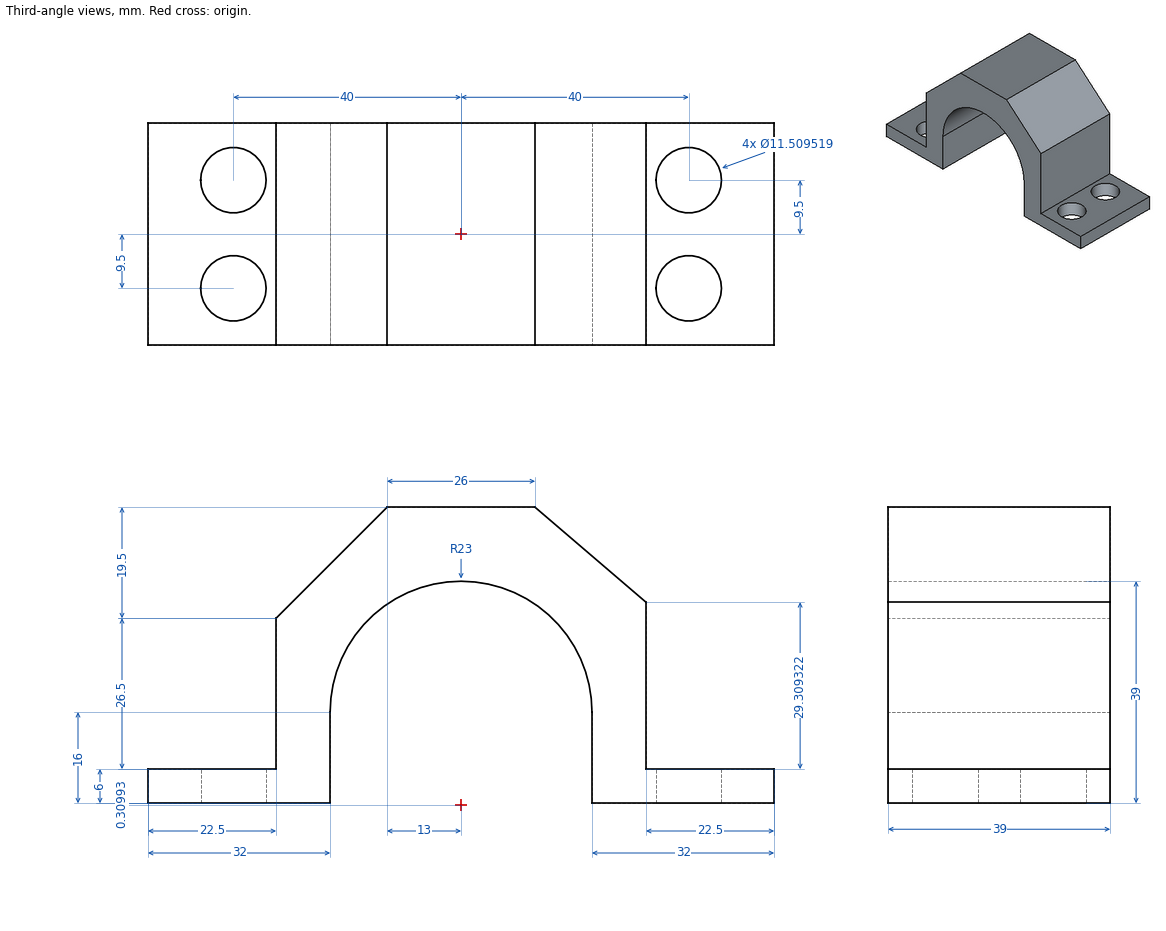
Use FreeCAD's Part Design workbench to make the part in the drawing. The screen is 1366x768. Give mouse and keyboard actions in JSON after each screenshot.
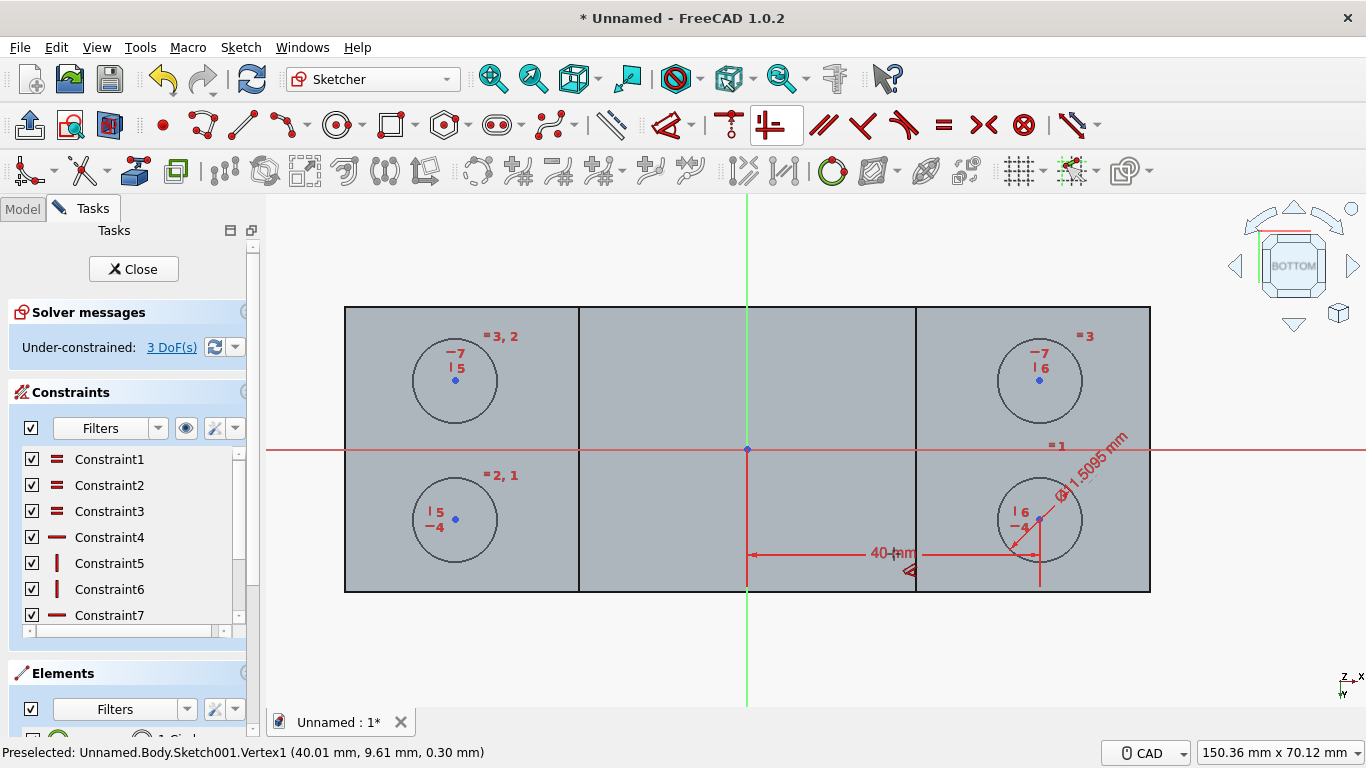
{"action": "left_click", "coordinate": [455, 520]}
{"action": "left_click", "coordinate": [601, 554]}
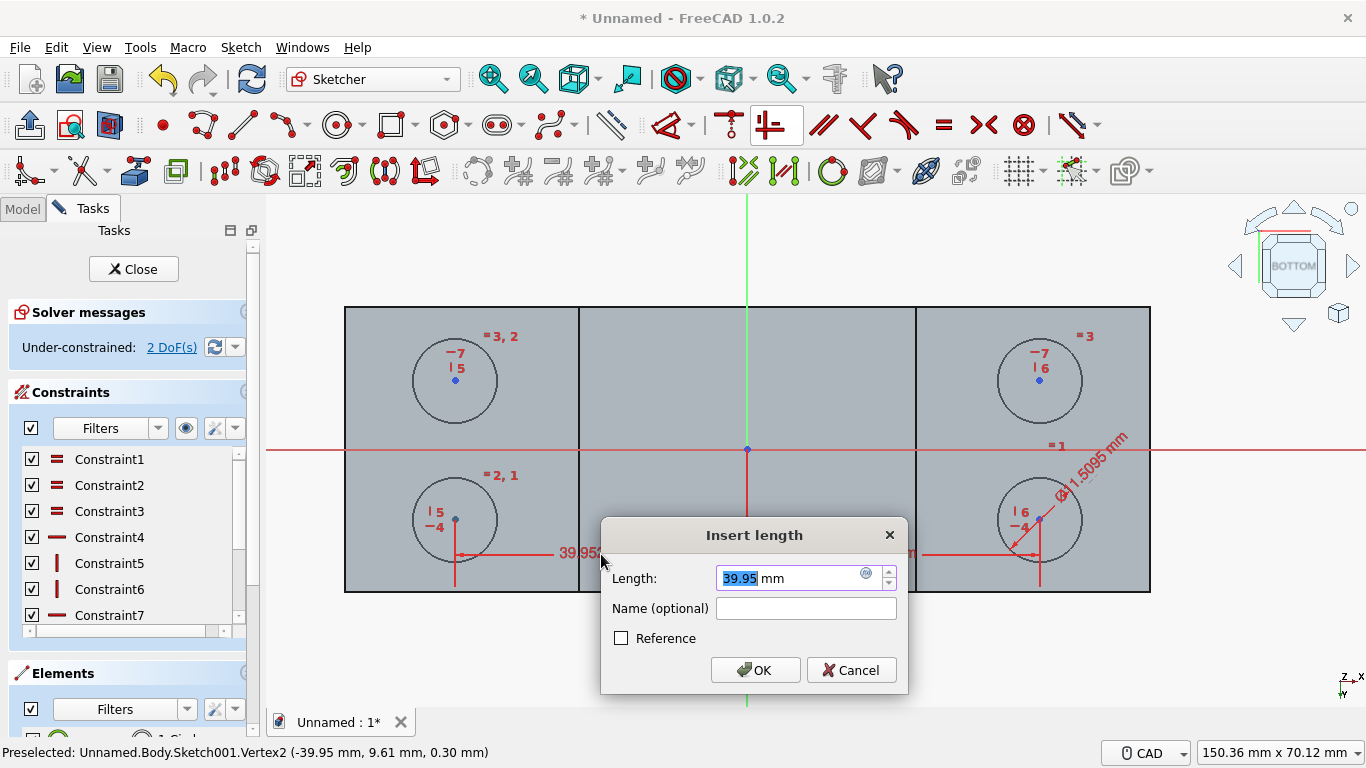
{"action": "type", "text": "40"}
{"action": "key", "text": "Return"}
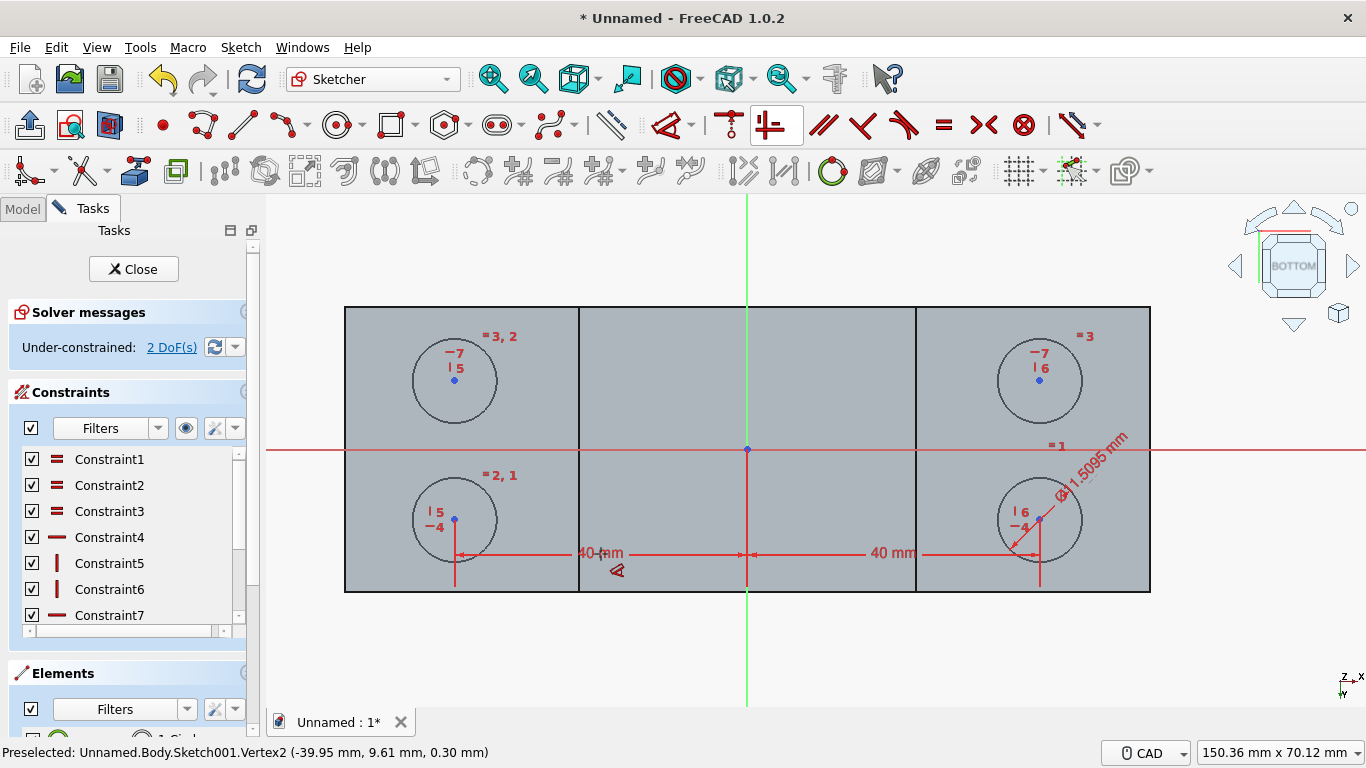
{"action": "left_click", "coordinate": [1040, 520]}
{"action": "left_click", "coordinate": [713, 485]}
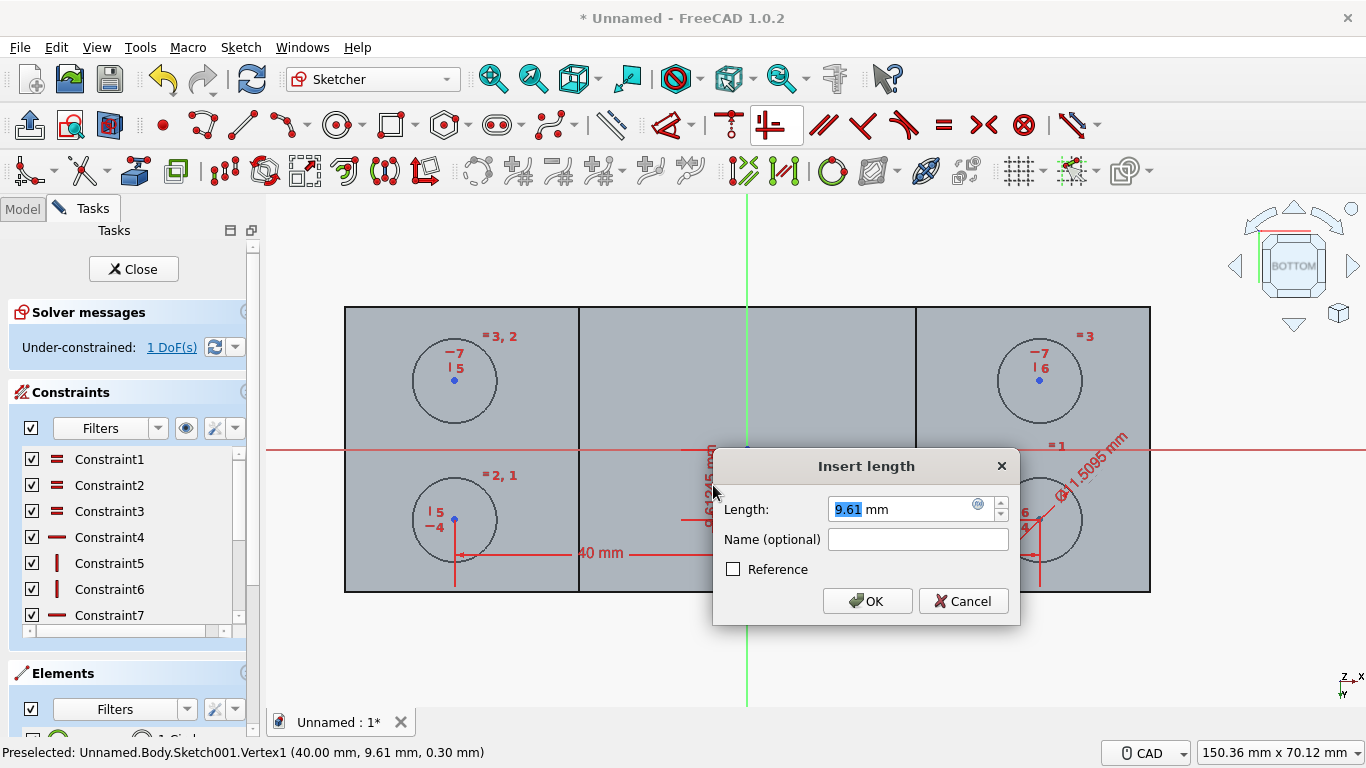
{"action": "type", "text": "9.5"}
{"action": "key", "text": "Return"}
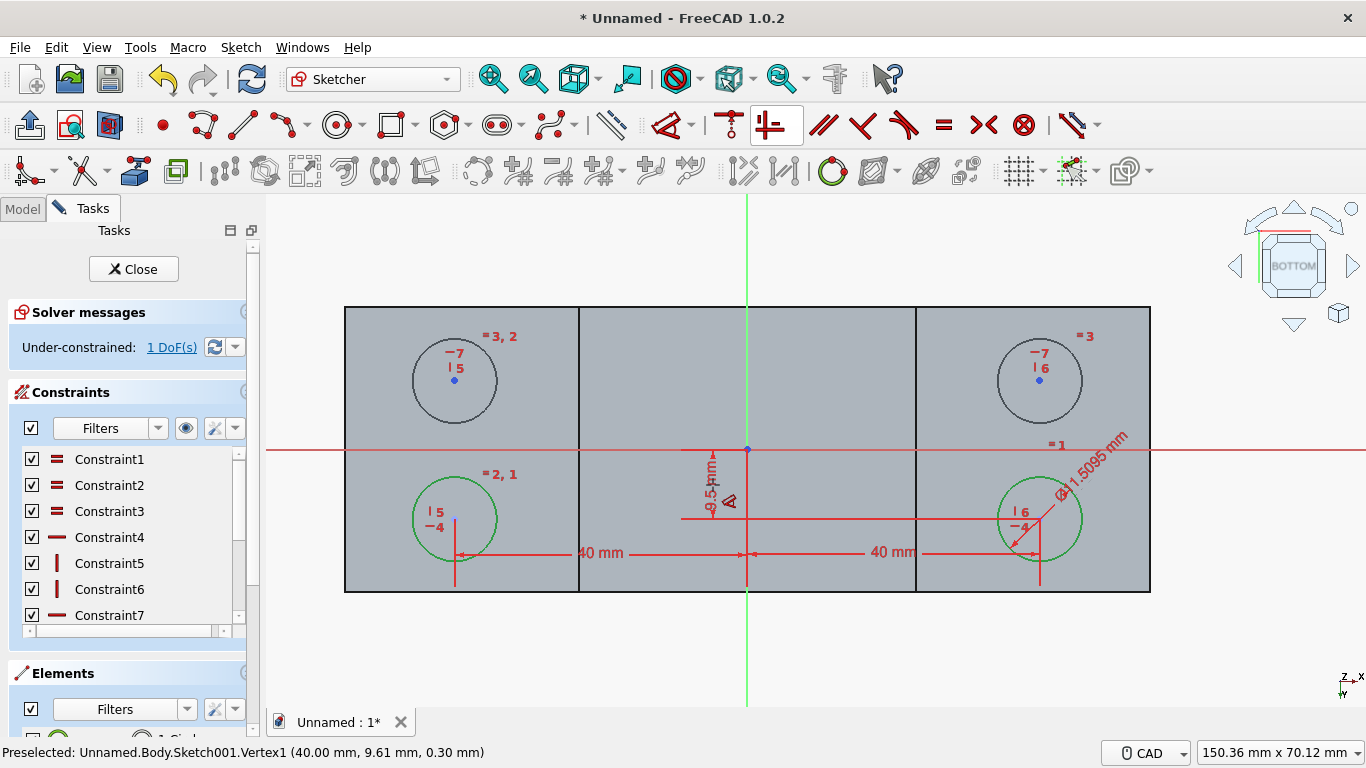
{"action": "left_click", "coordinate": [455, 381]}
{"action": "left_click", "coordinate": [421, 431]}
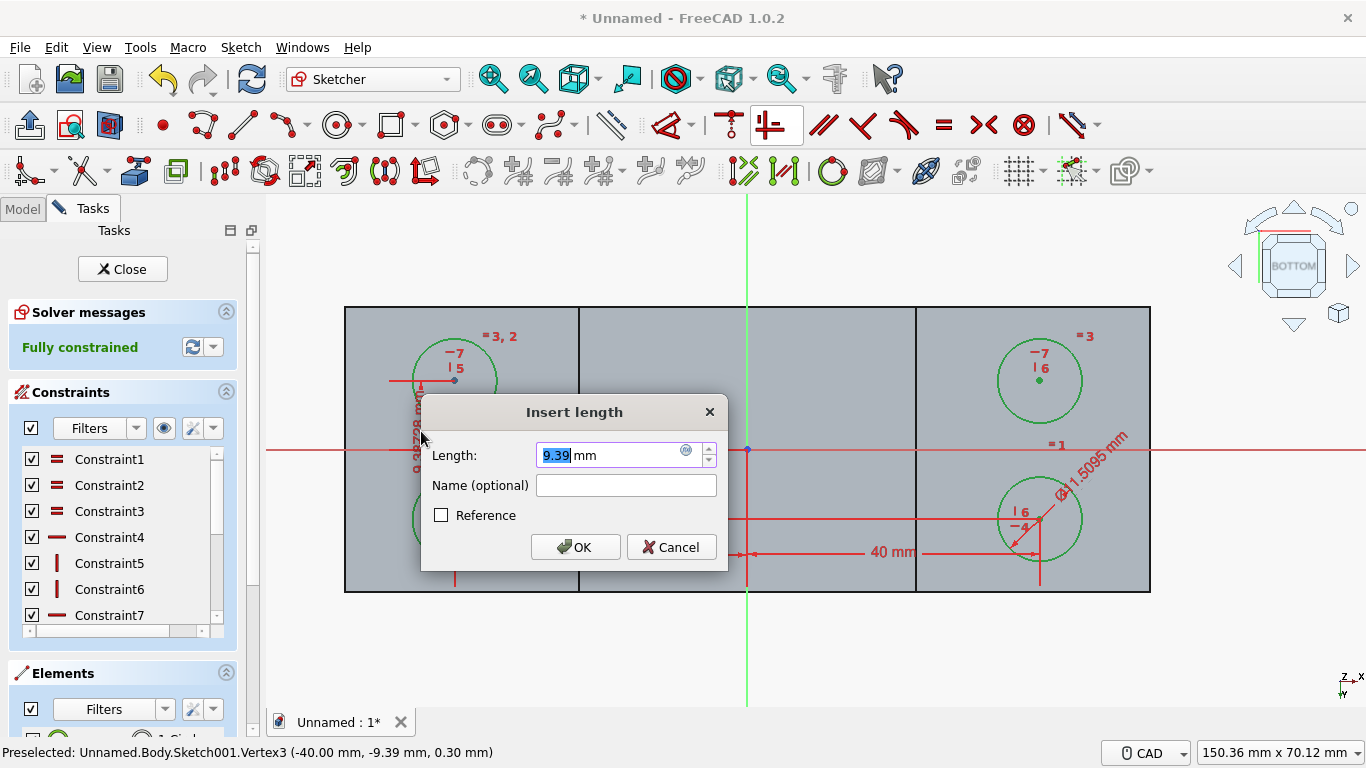
{"action": "type", "text": "9.5"}
{"action": "key", "text": "Return"}
{"action": "key", "text": "Escape"}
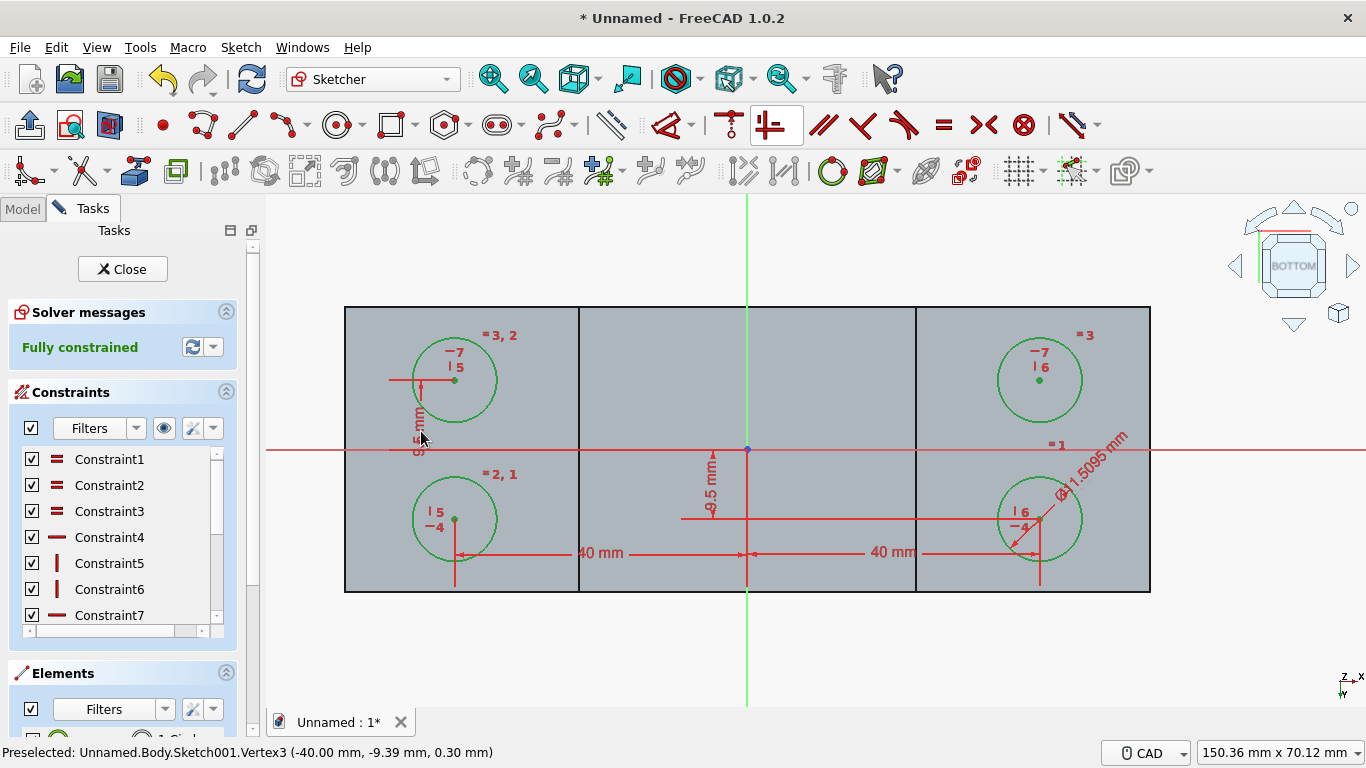
{"action": "left_click", "coordinate": [123, 269]}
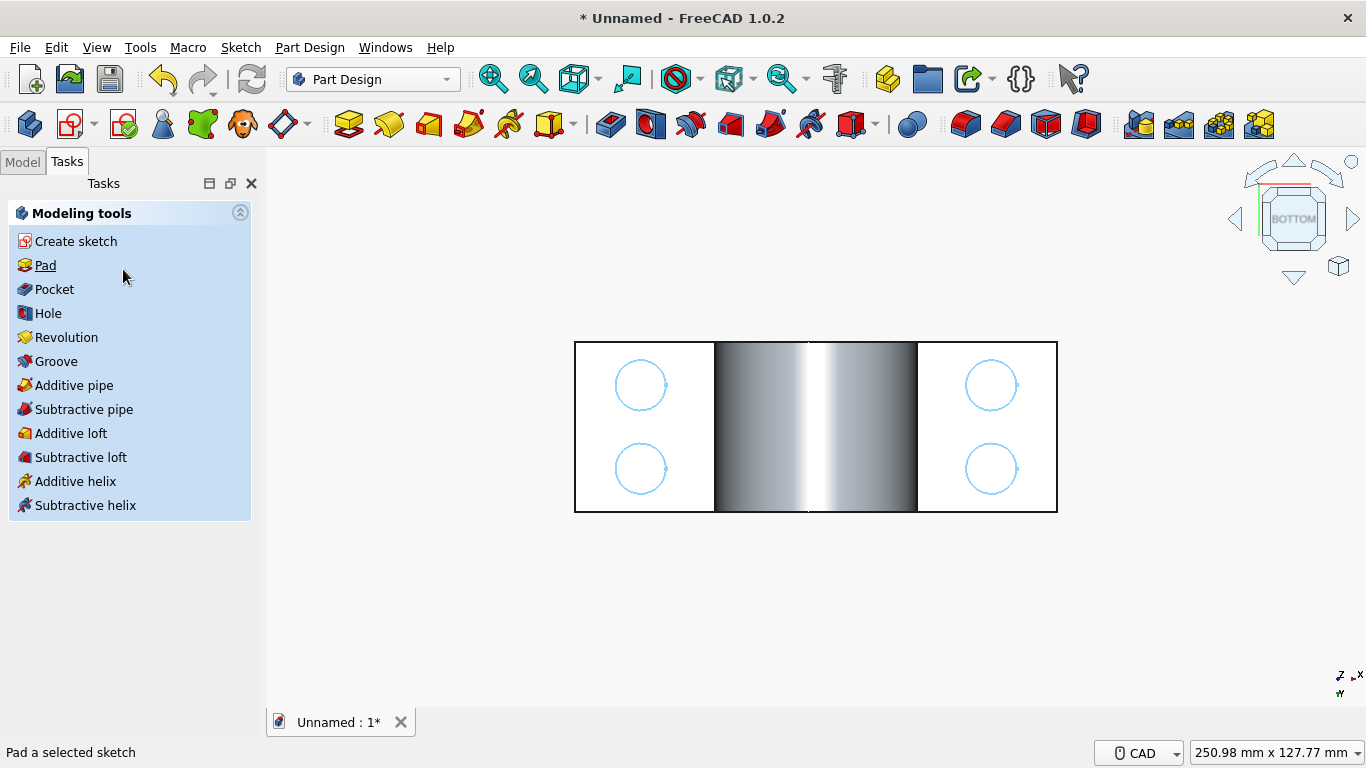
{"action": "left_click", "coordinate": [612, 124]}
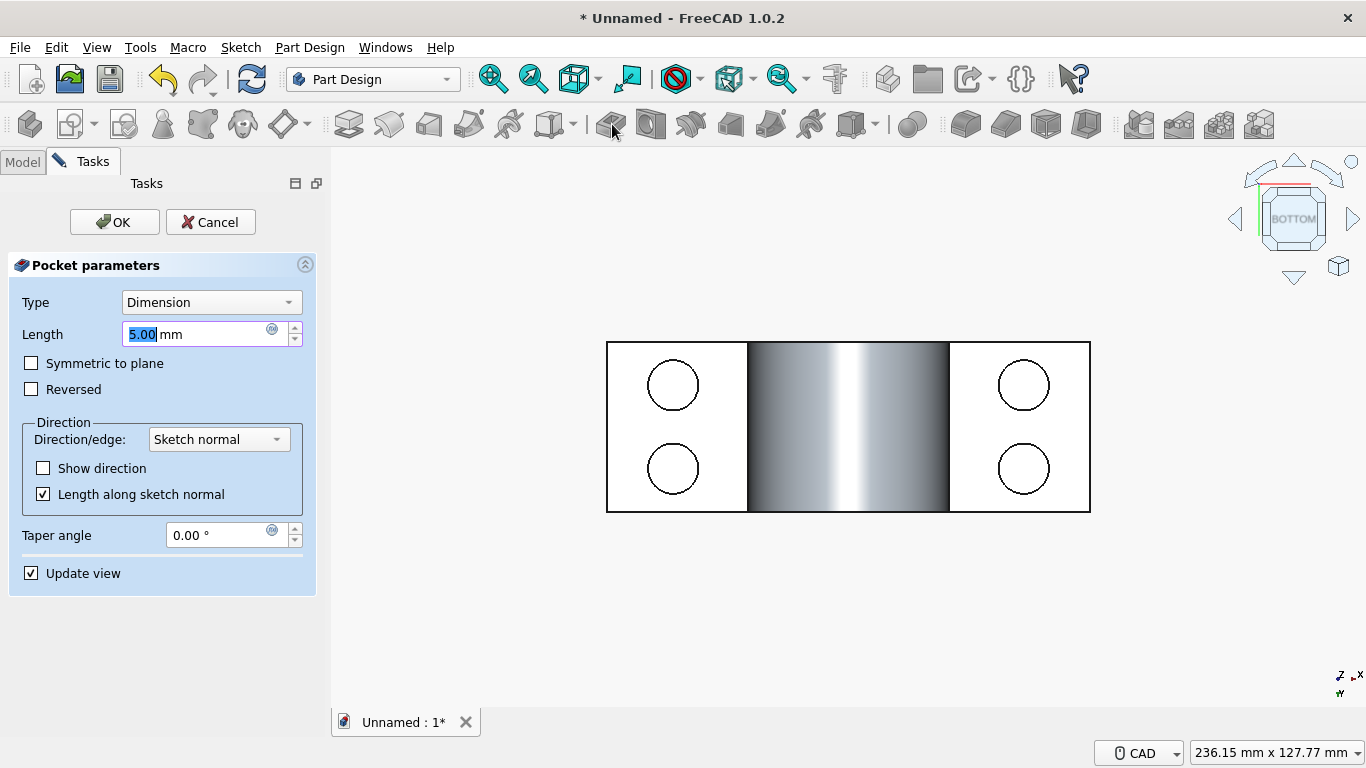
{"action": "type", "text": "39"}
{"action": "key", "text": "Tab"}